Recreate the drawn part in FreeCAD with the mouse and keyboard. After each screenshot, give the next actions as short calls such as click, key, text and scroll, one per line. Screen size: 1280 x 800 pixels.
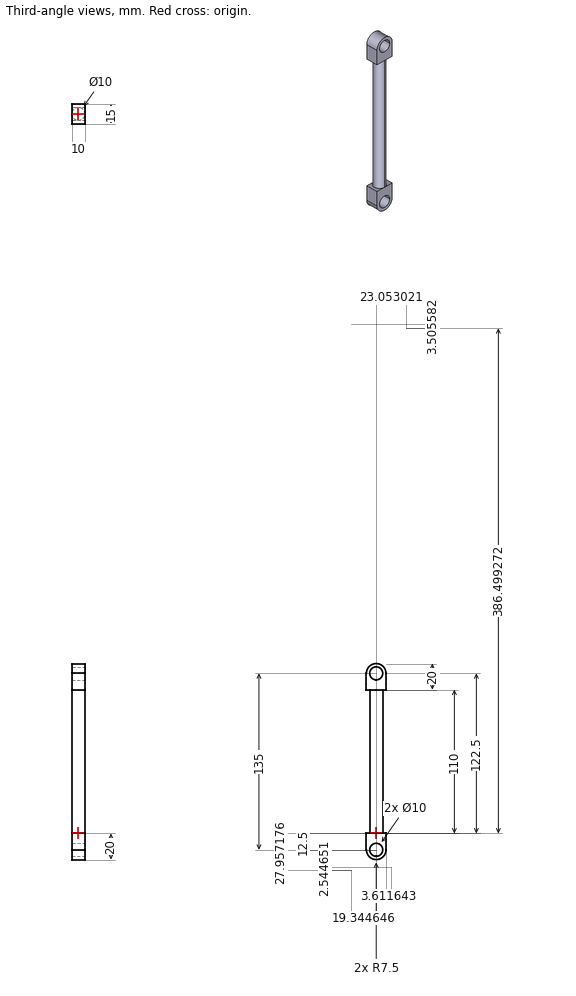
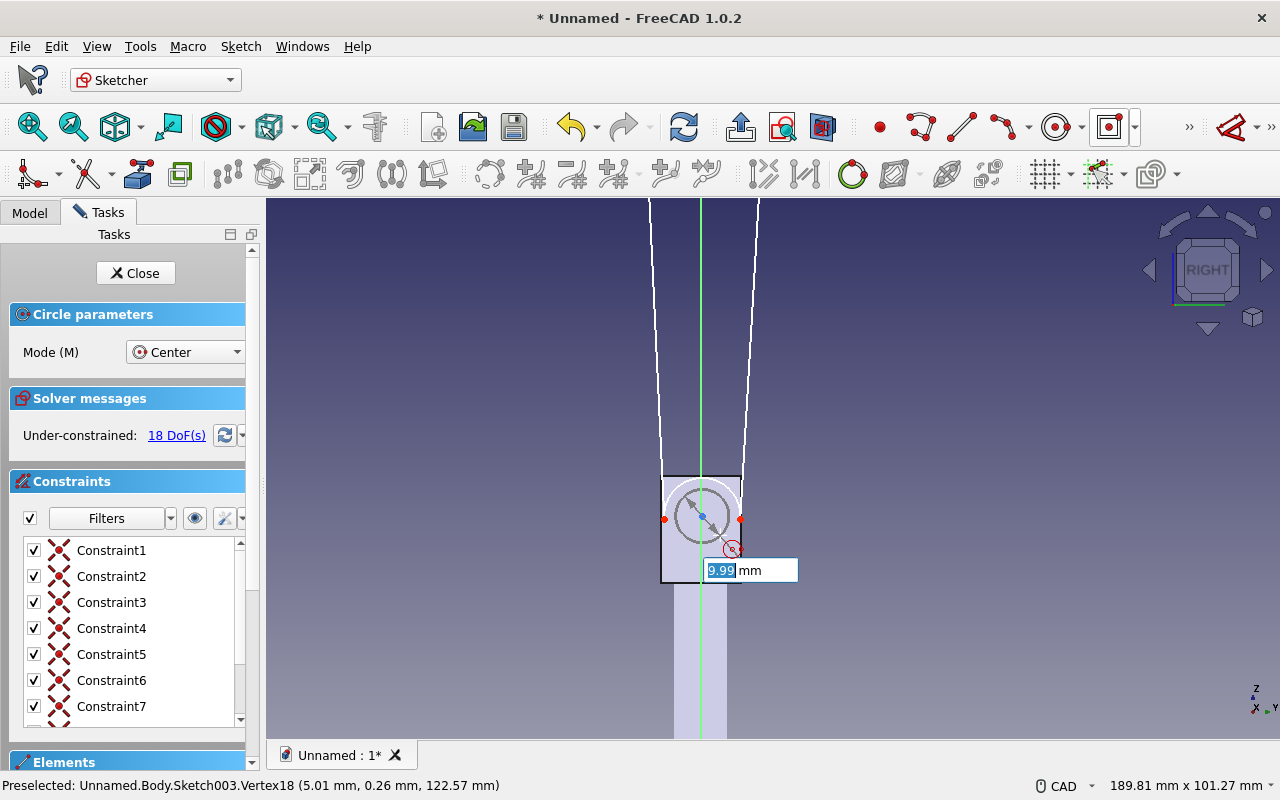
text(10)
key(Return)
key(Escape)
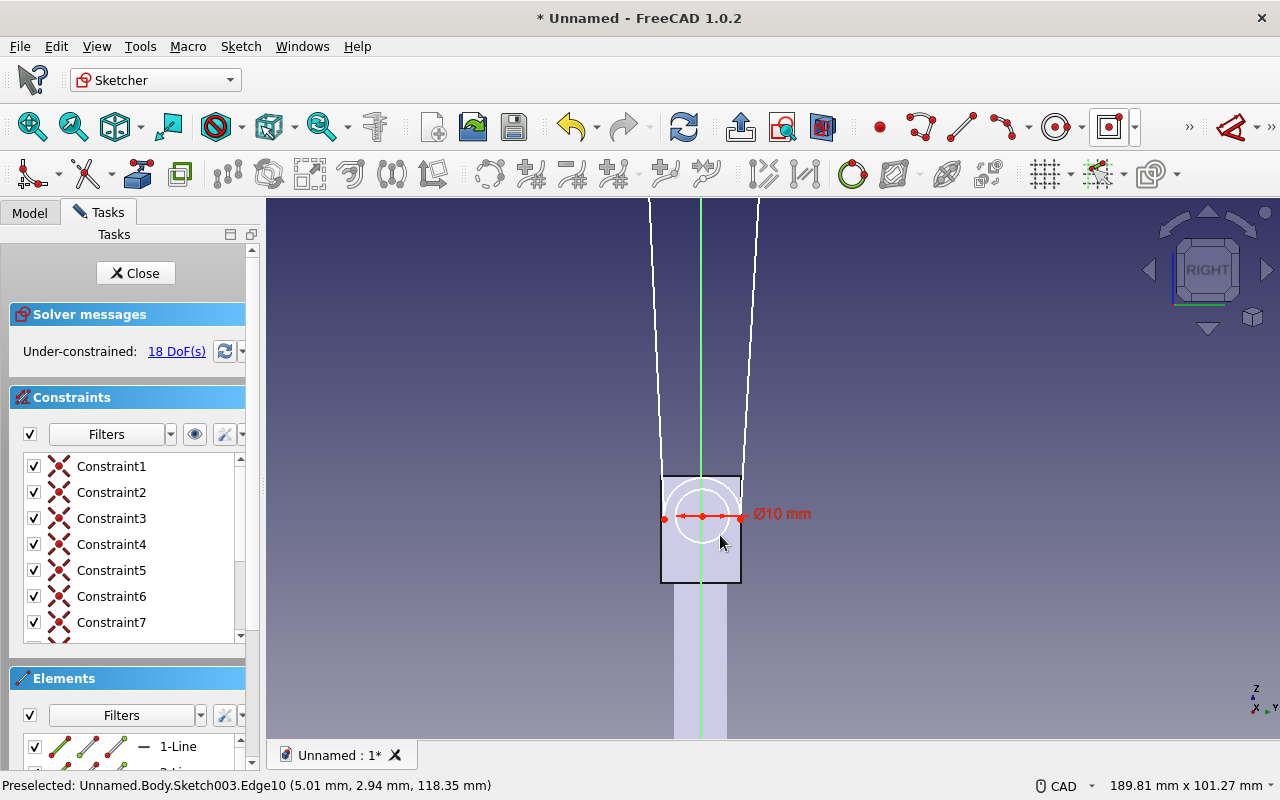
scroll(703, 521, down, 9)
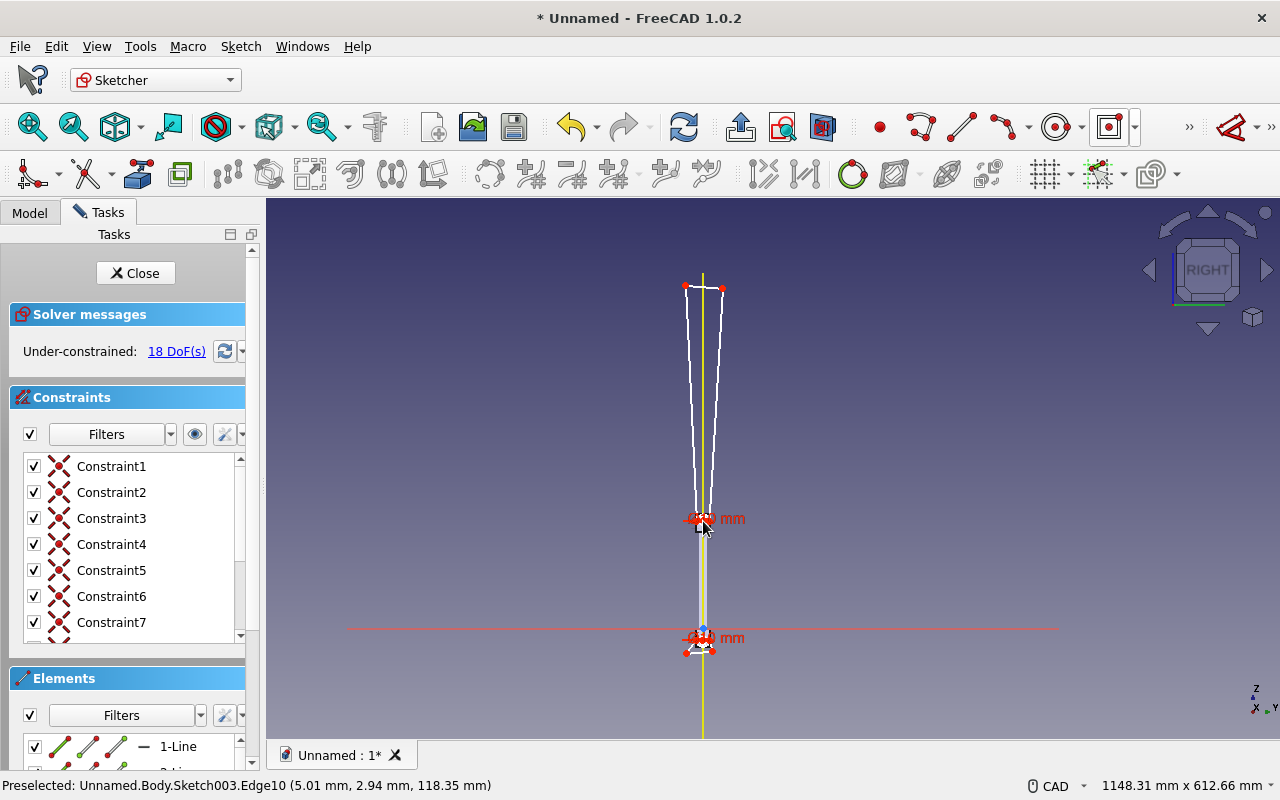
scroll(699, 646, up, 10)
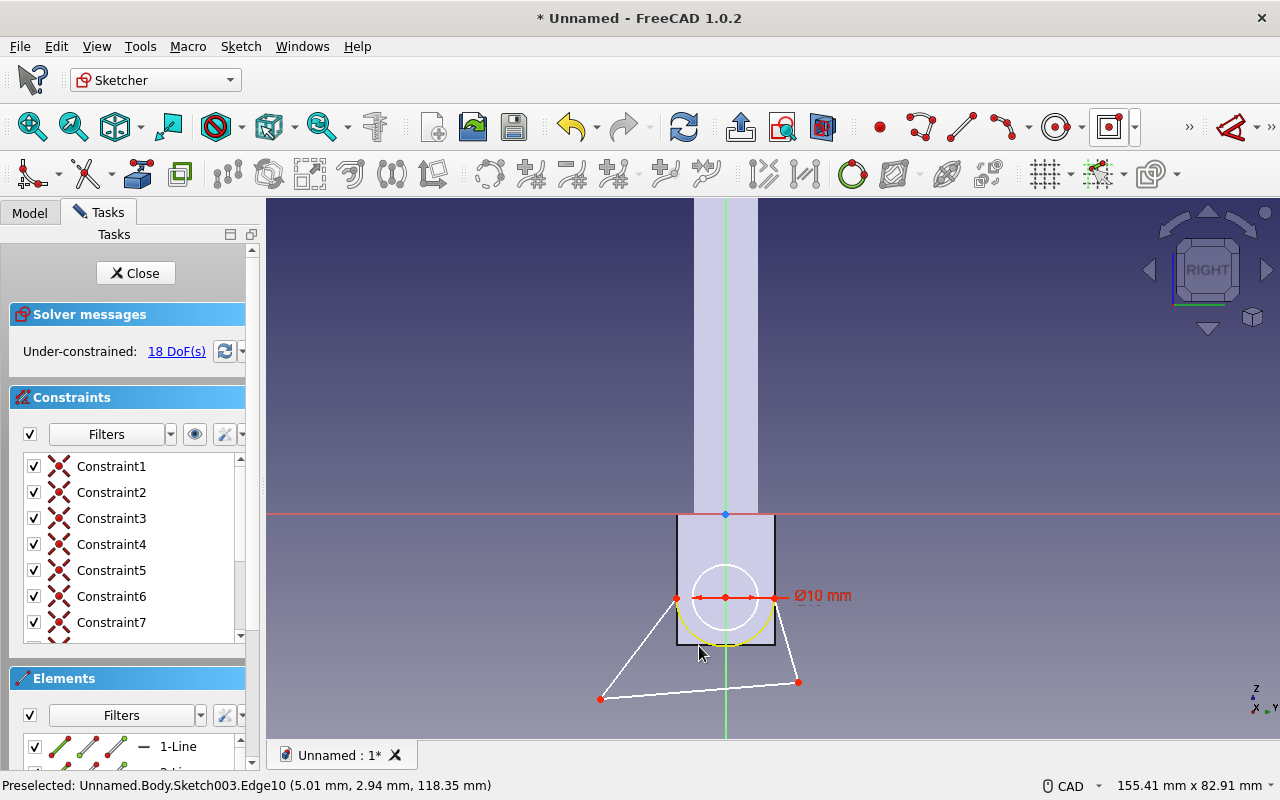
click(697, 637)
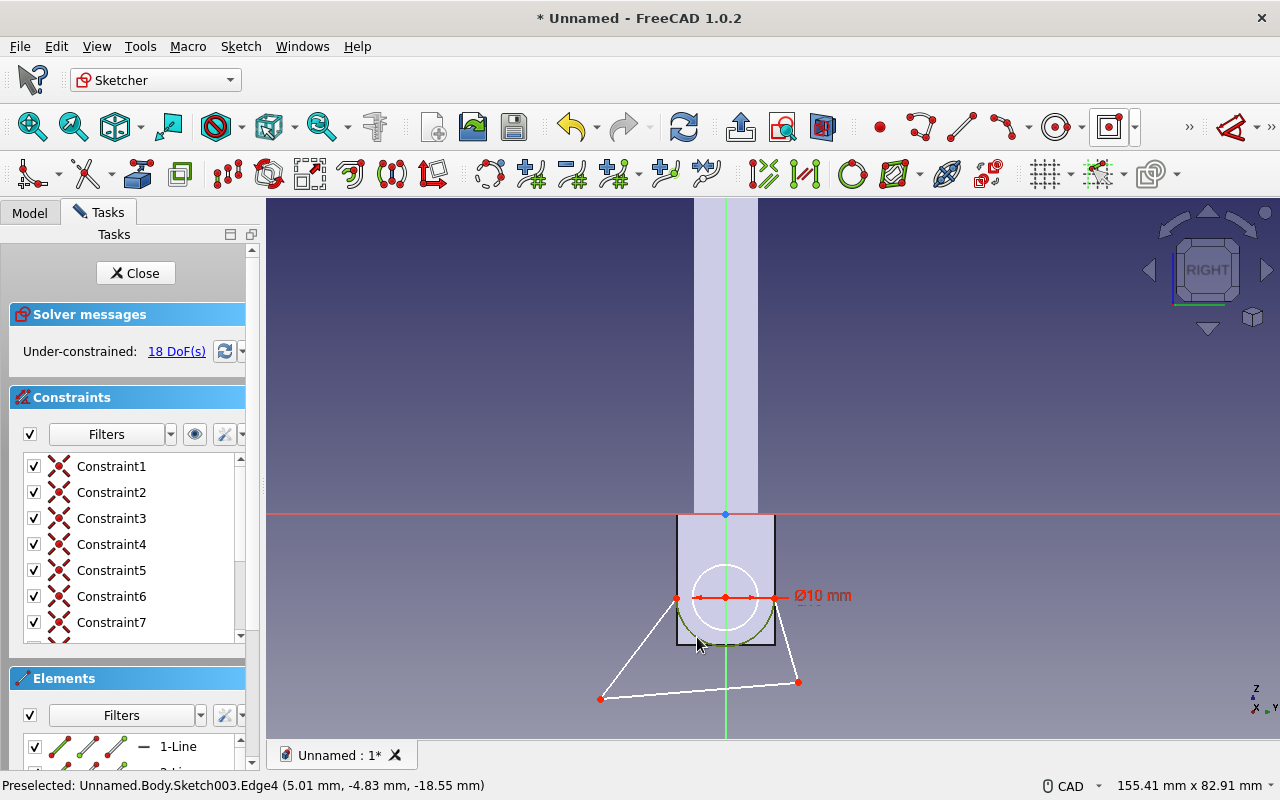
scroll(699, 646, down, 10)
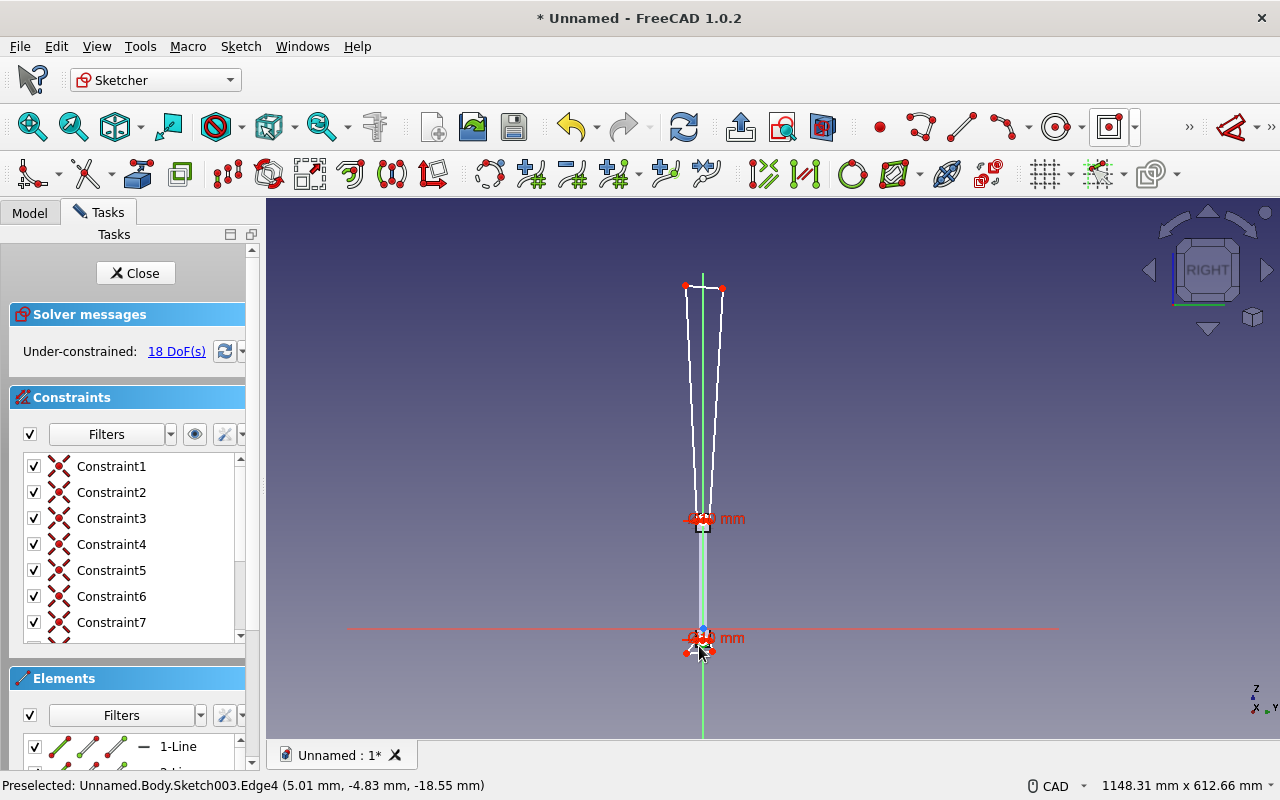
scroll(707, 516, up, 10)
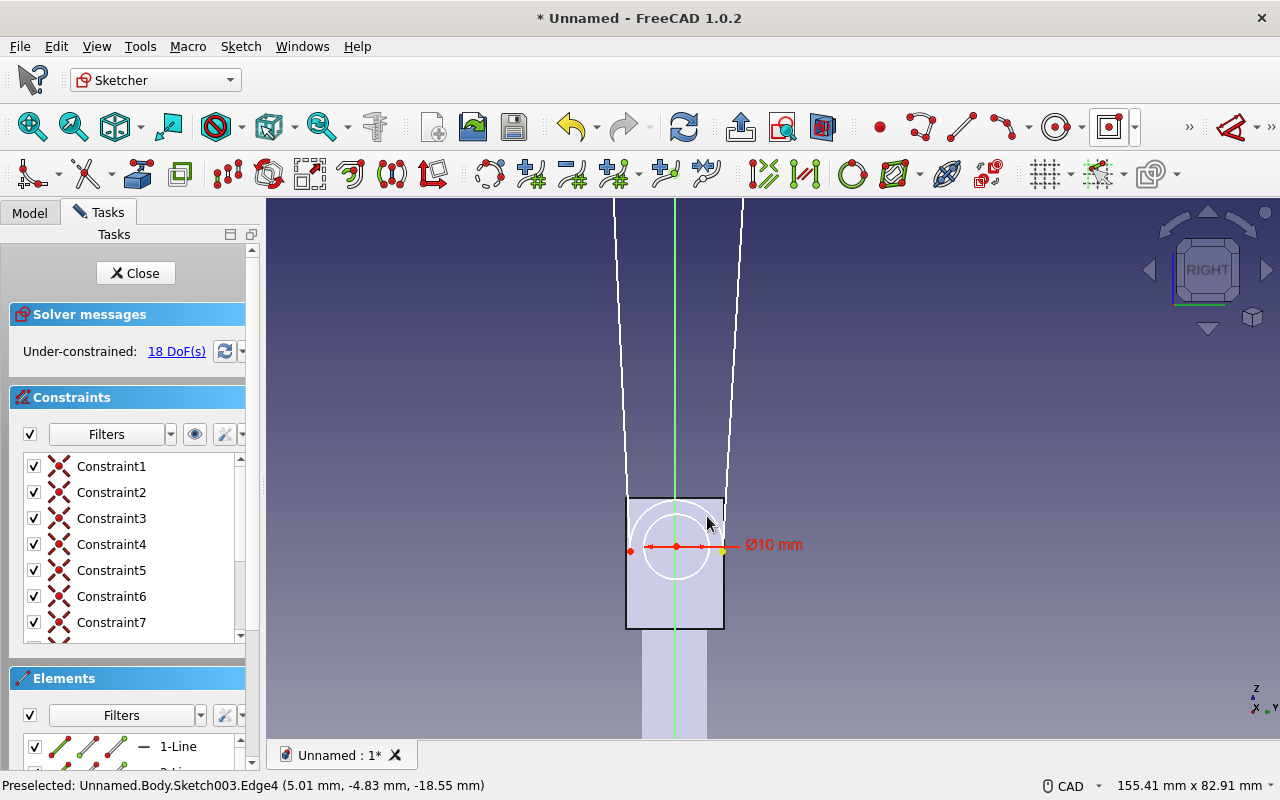
click(705, 510)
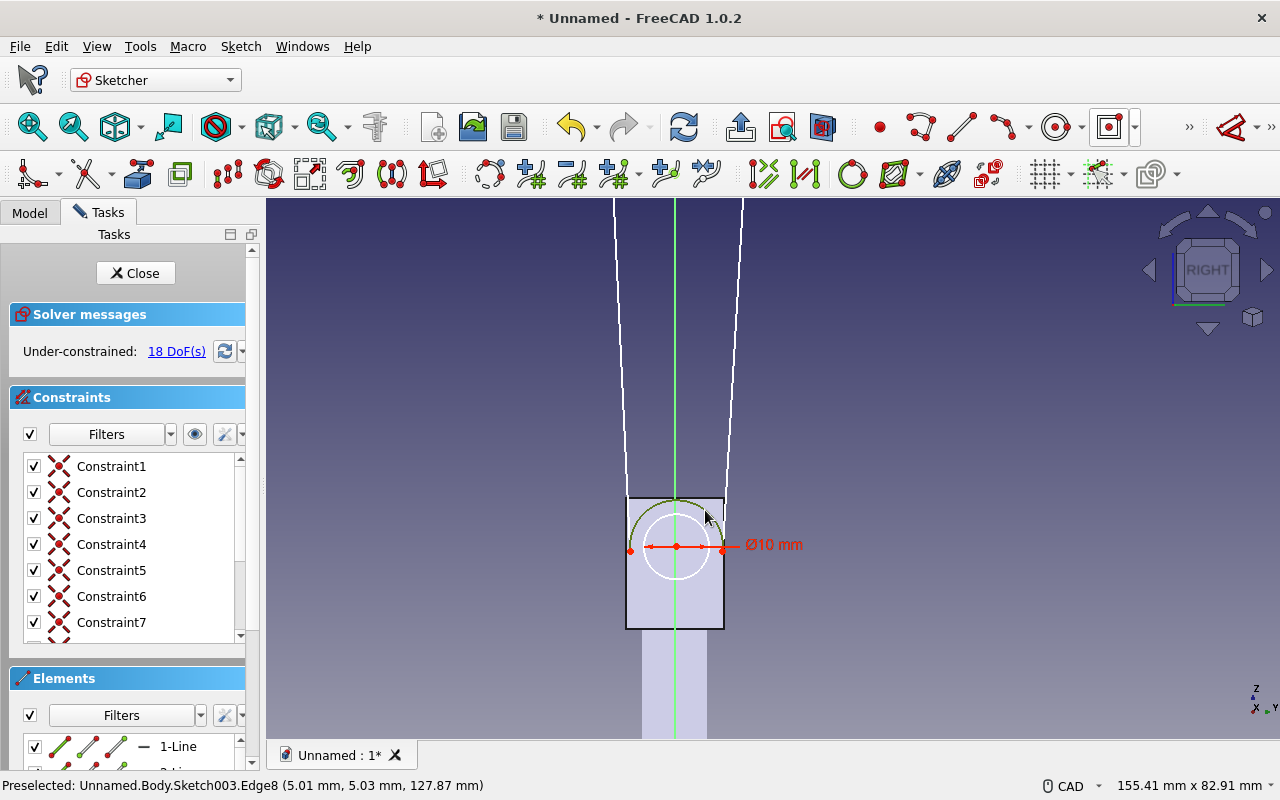
key(e)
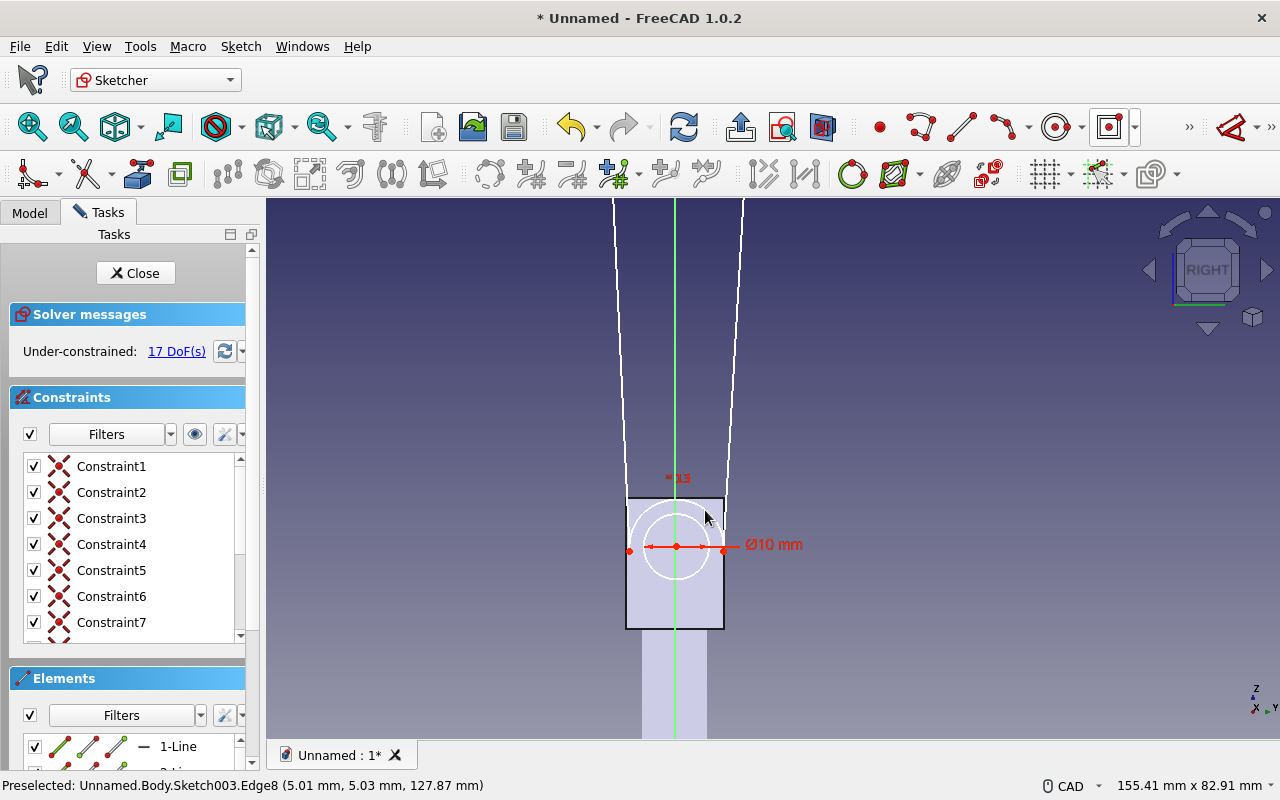
scroll(707, 516, down, 10)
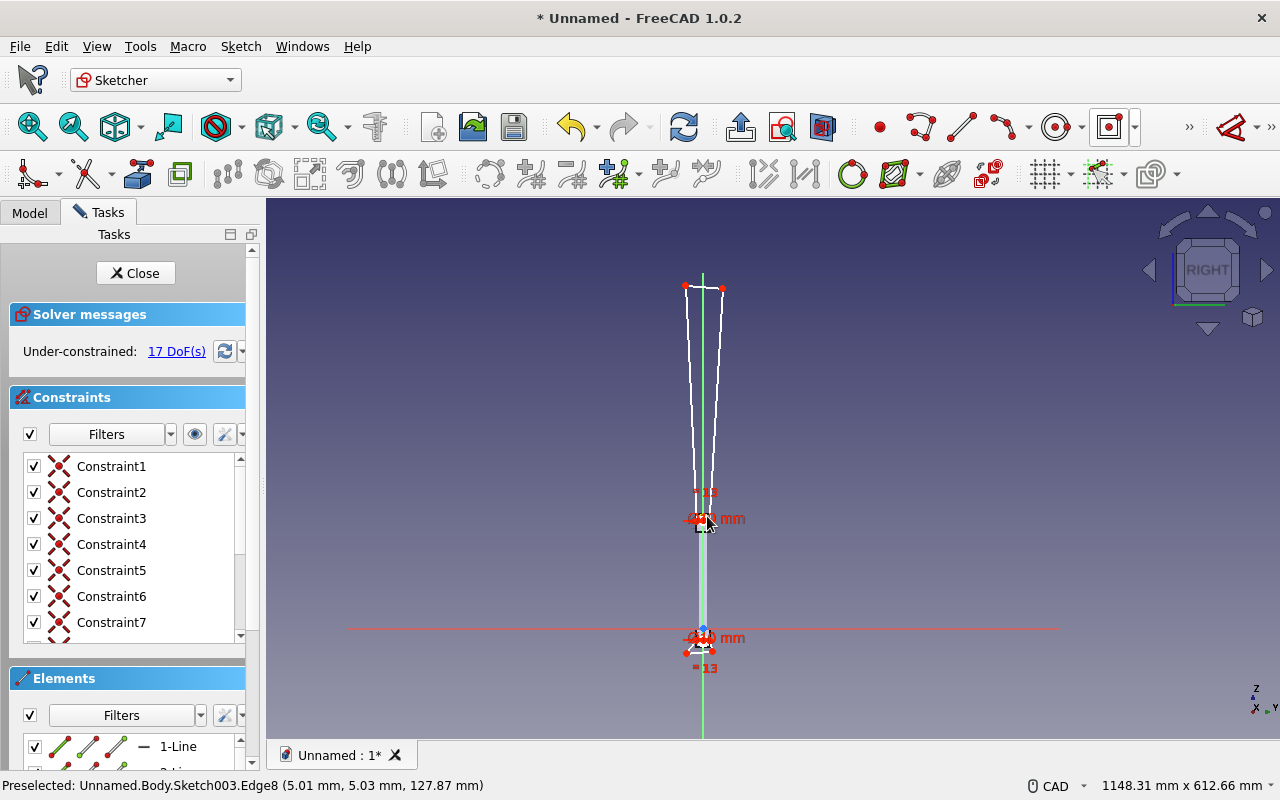
scroll(703, 640, up, 4)